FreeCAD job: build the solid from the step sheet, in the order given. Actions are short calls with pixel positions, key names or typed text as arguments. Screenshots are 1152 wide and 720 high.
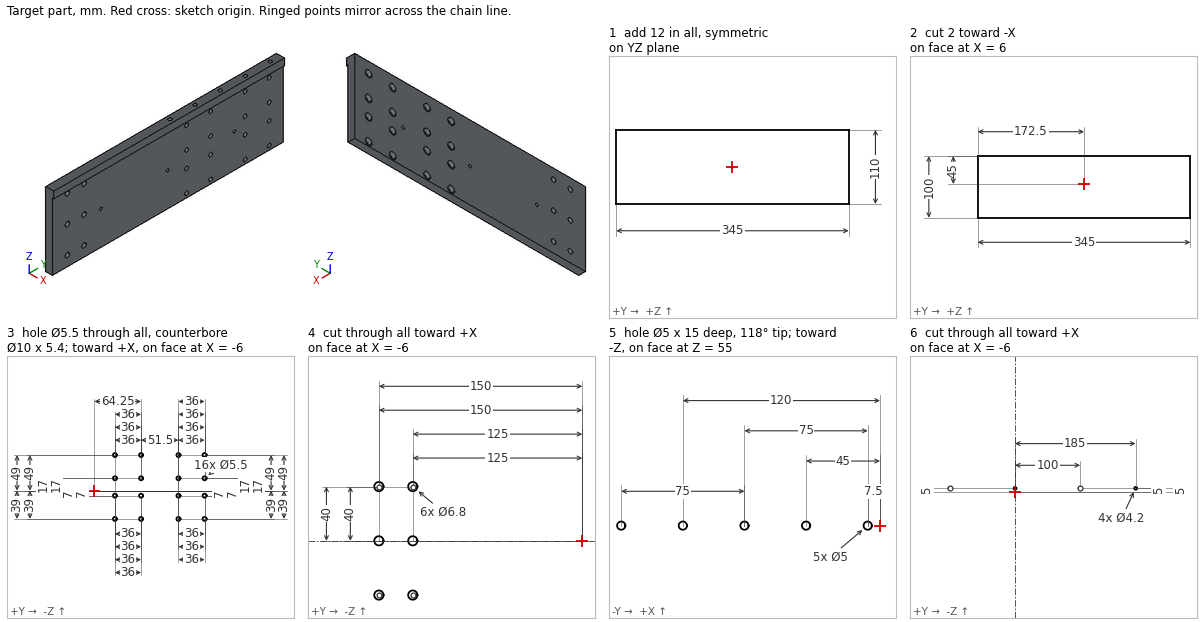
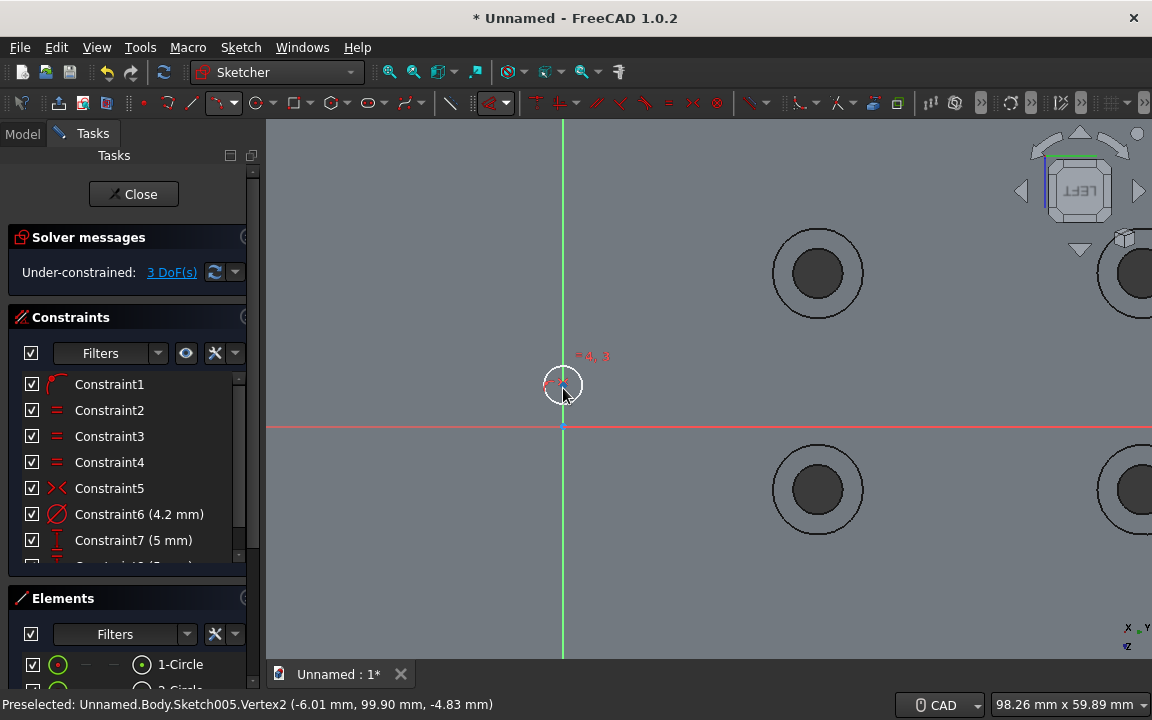
click(563, 385)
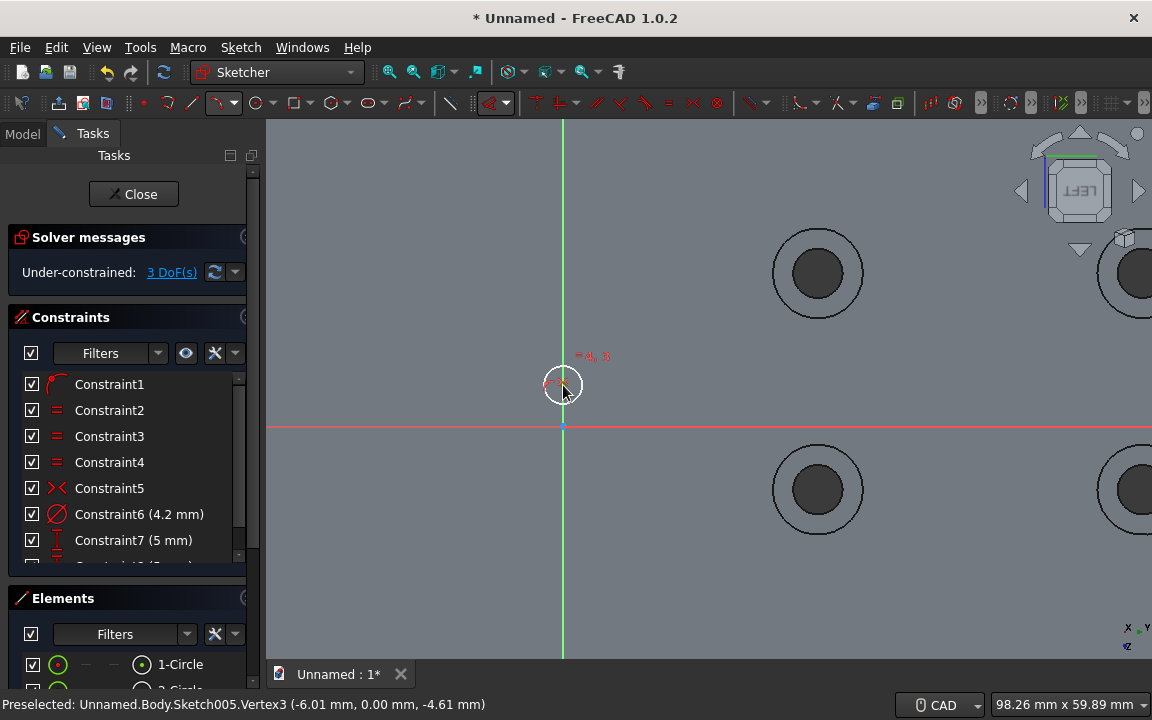
key(i)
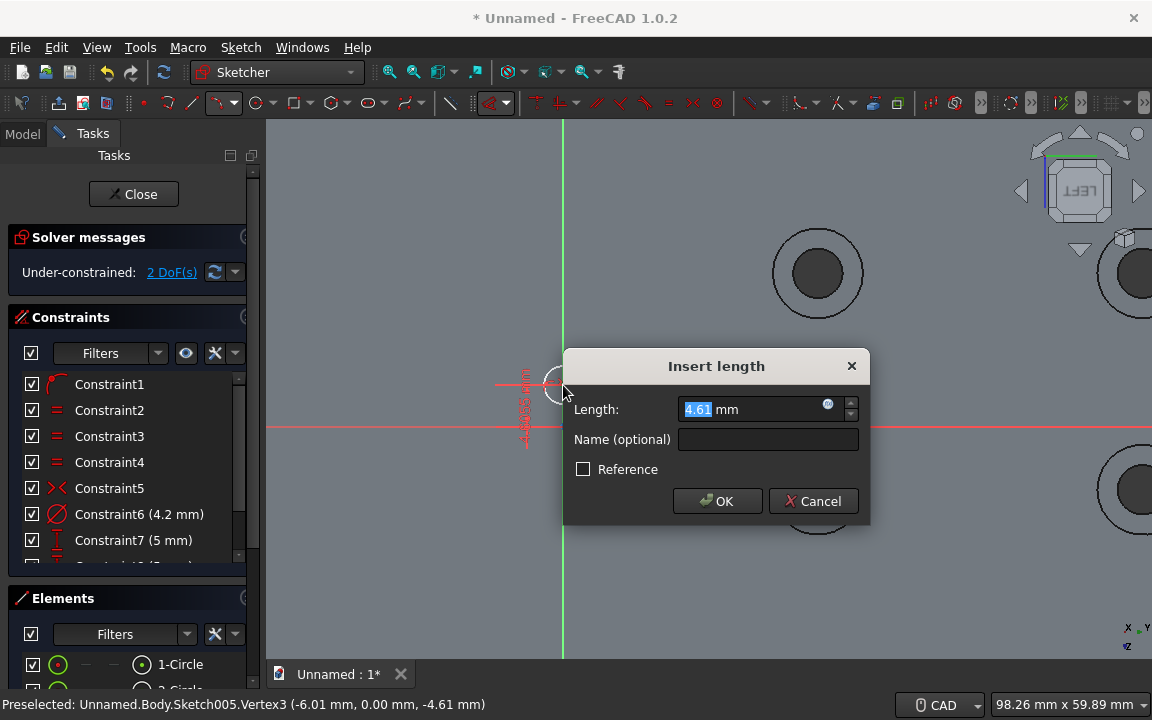
text(5)
key(Return)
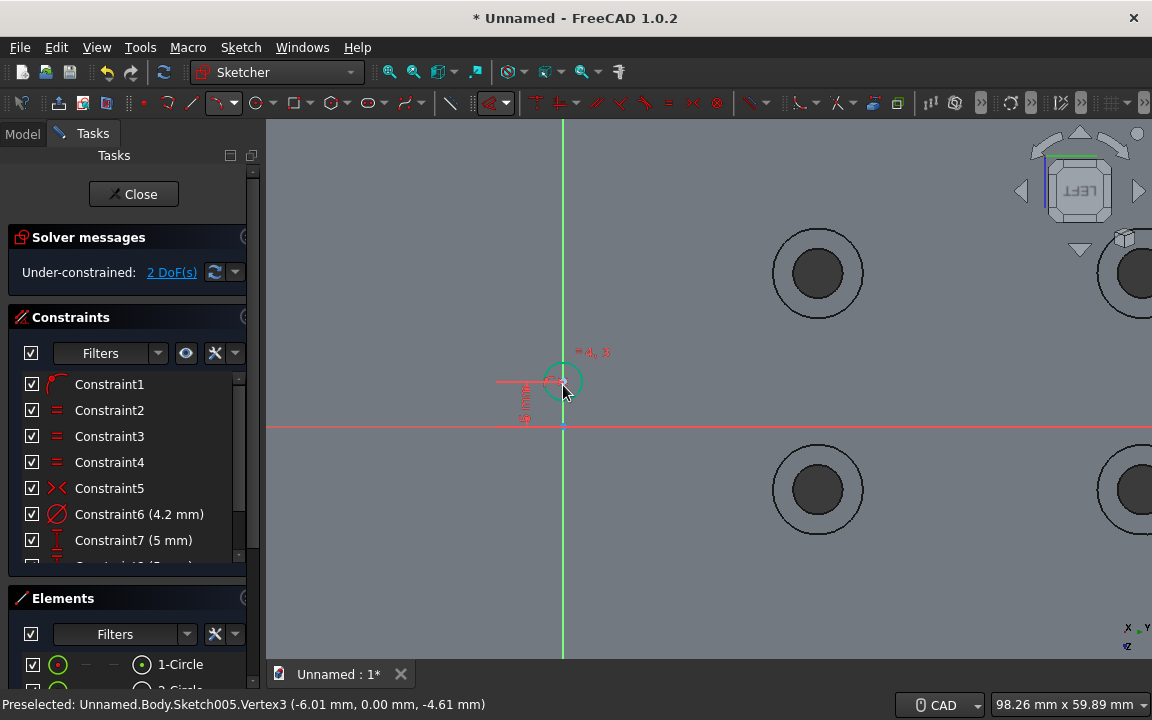
scroll(563, 388, down, 8)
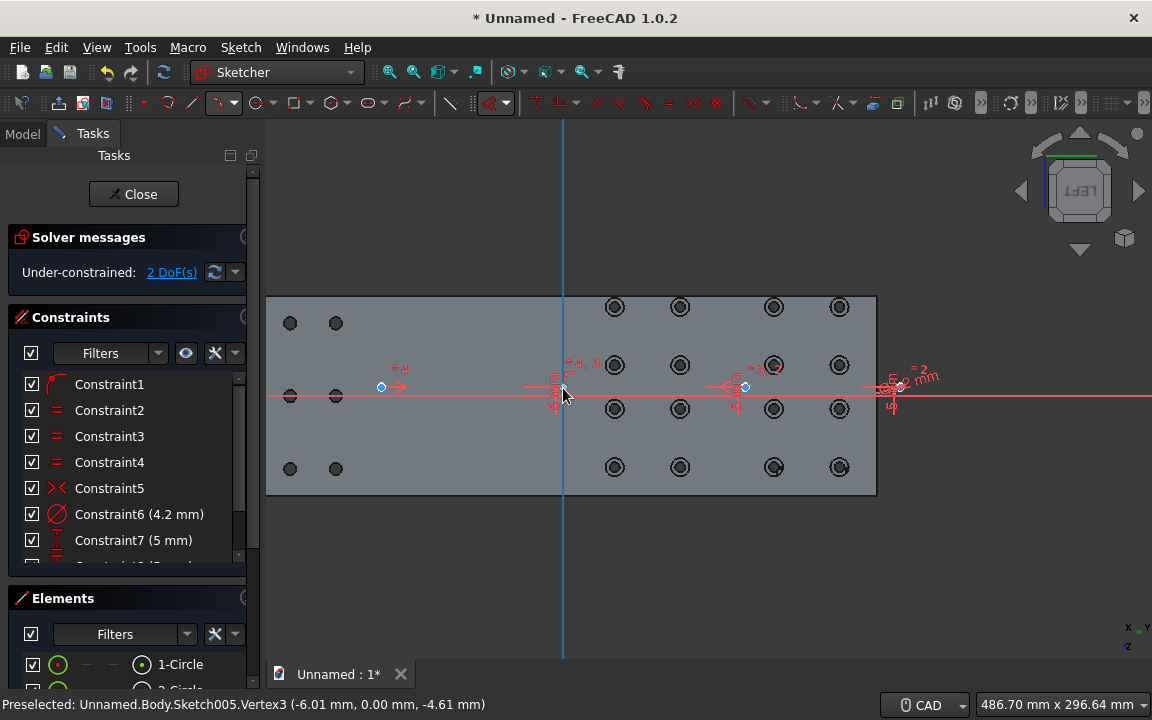
click(900, 387)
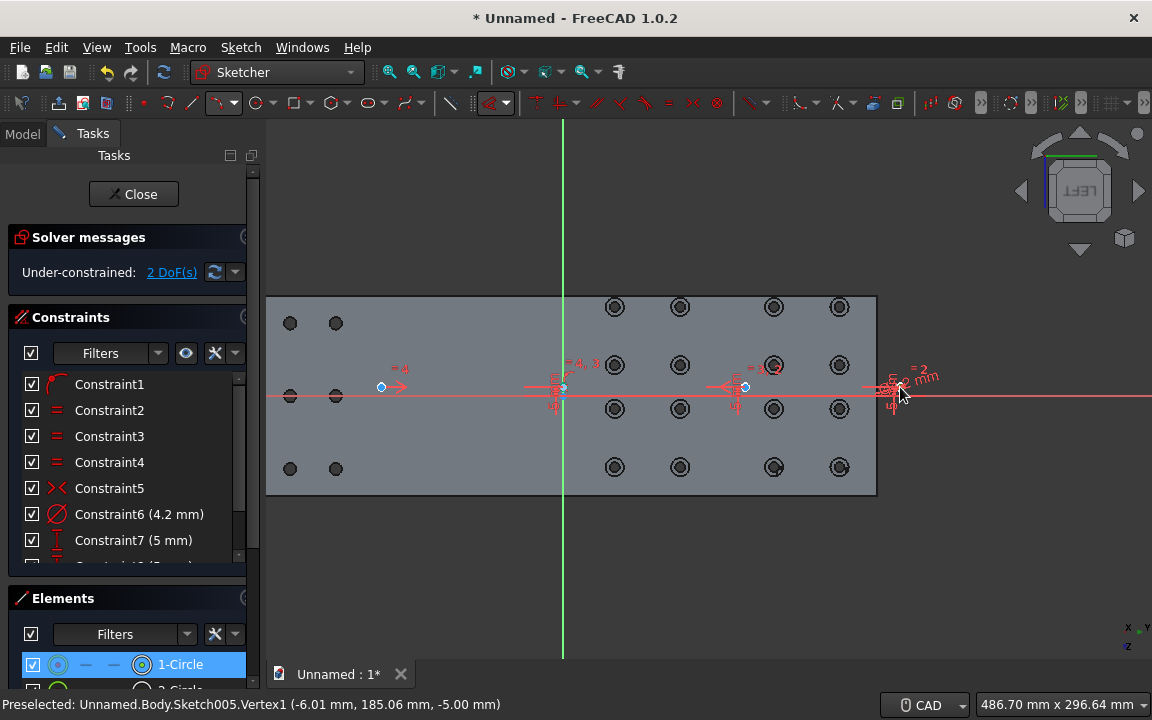
click(508, 104)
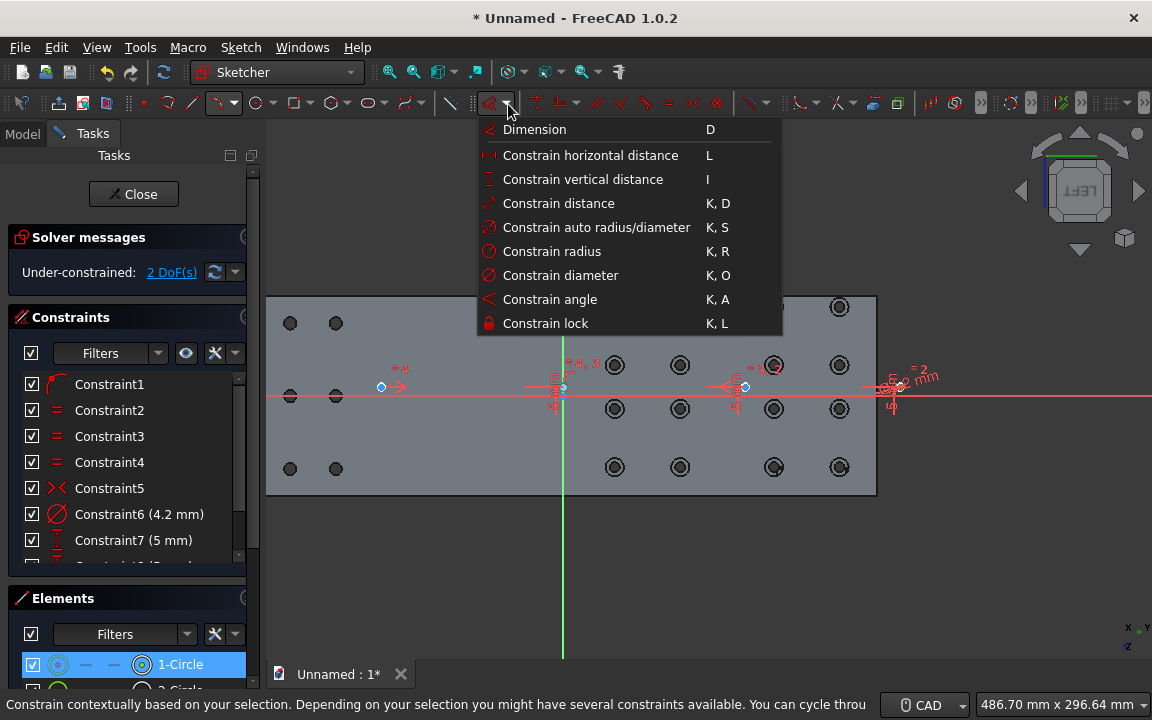
click(630, 155)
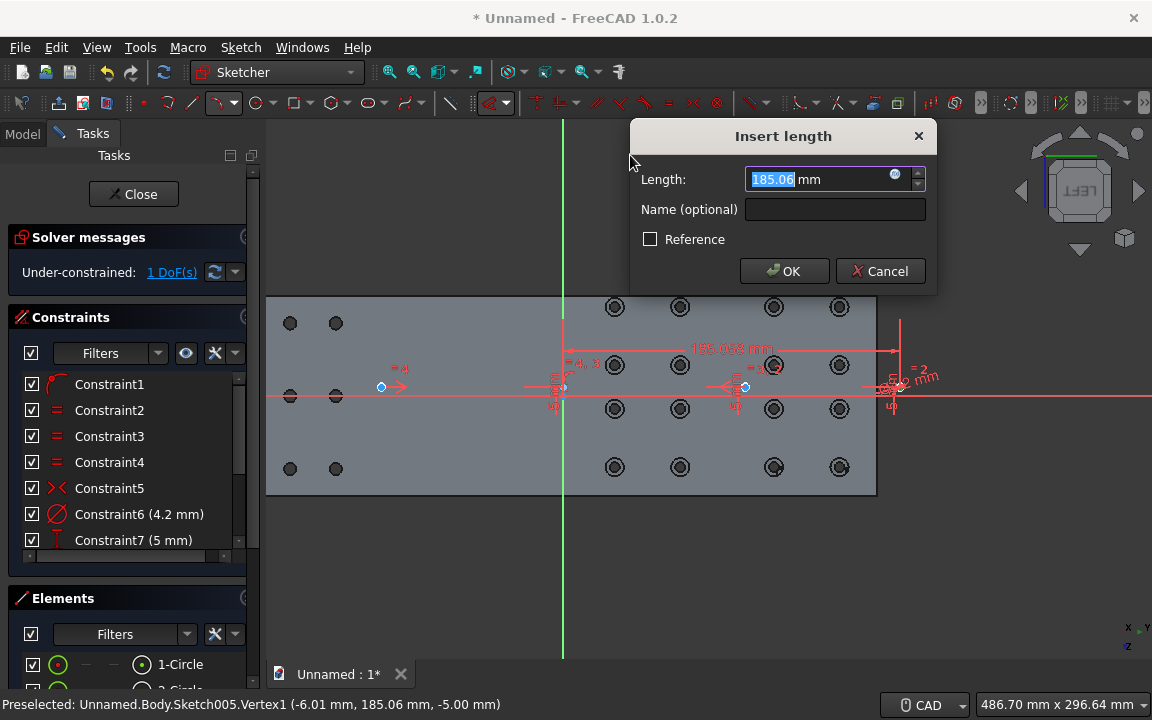
text(185)
key(Return)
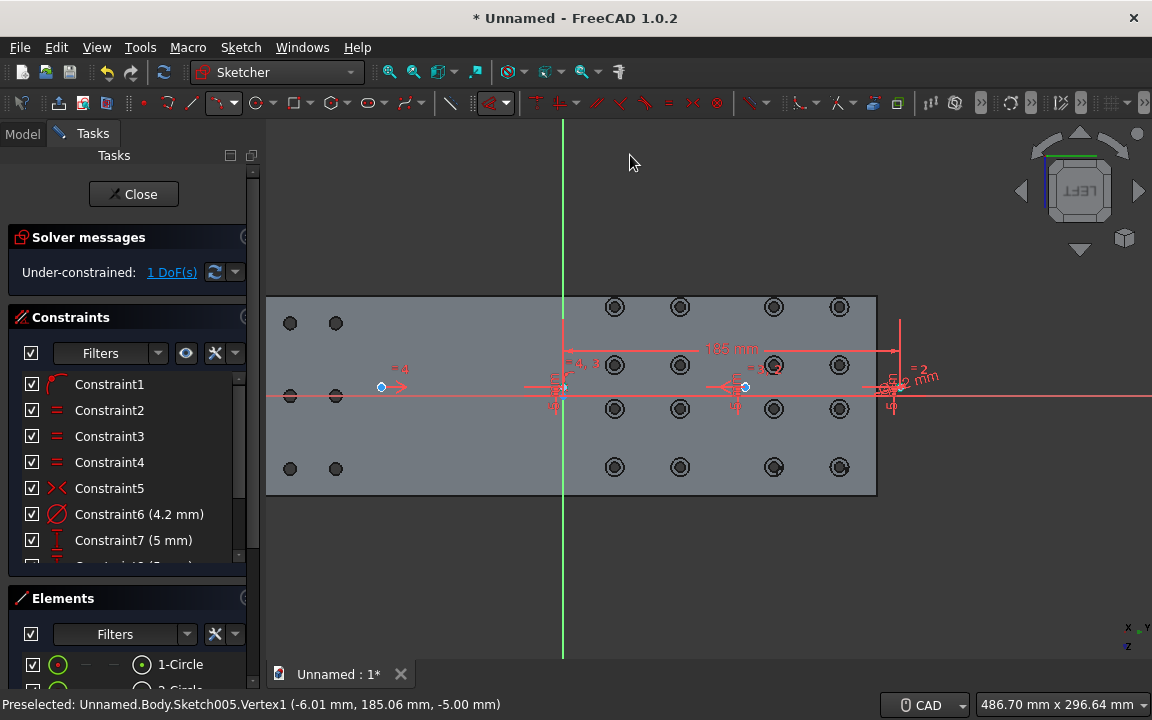
click(745, 387)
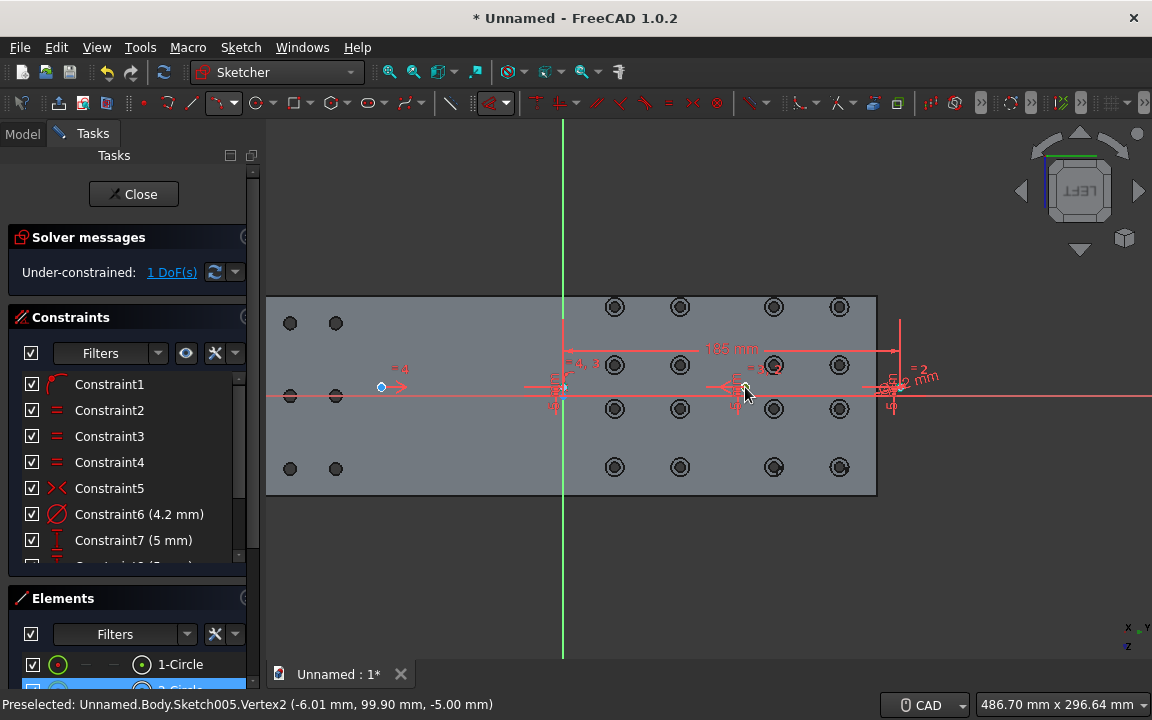
click(508, 104)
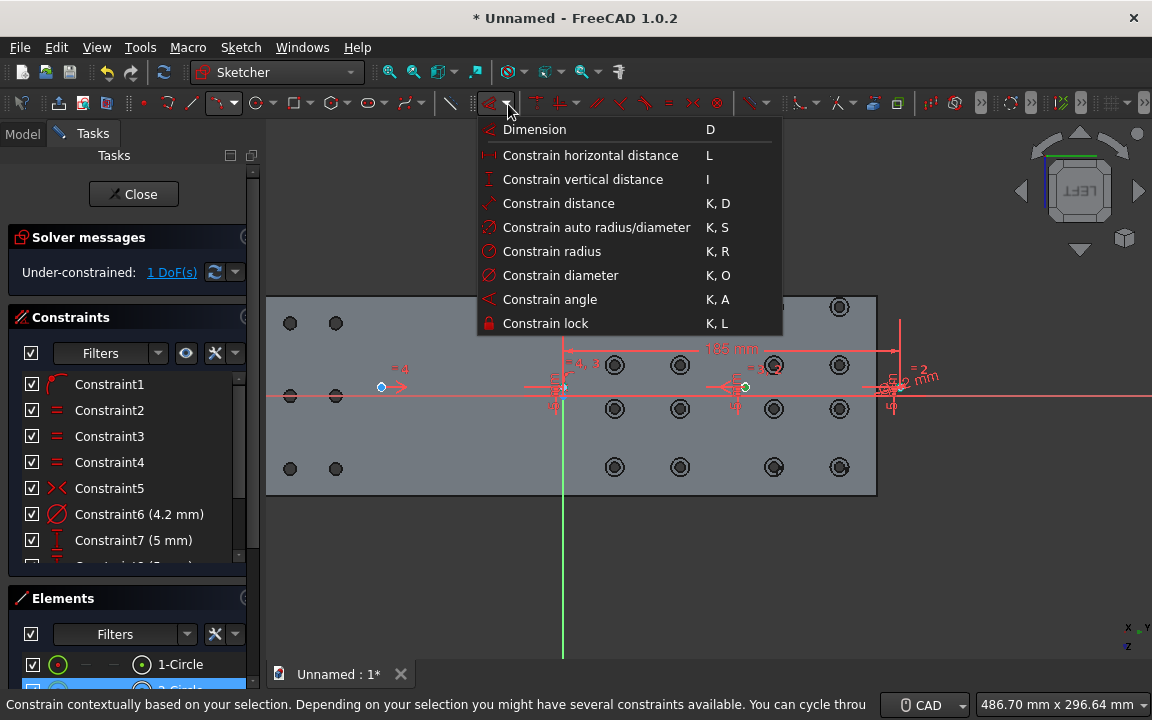
click(630, 155)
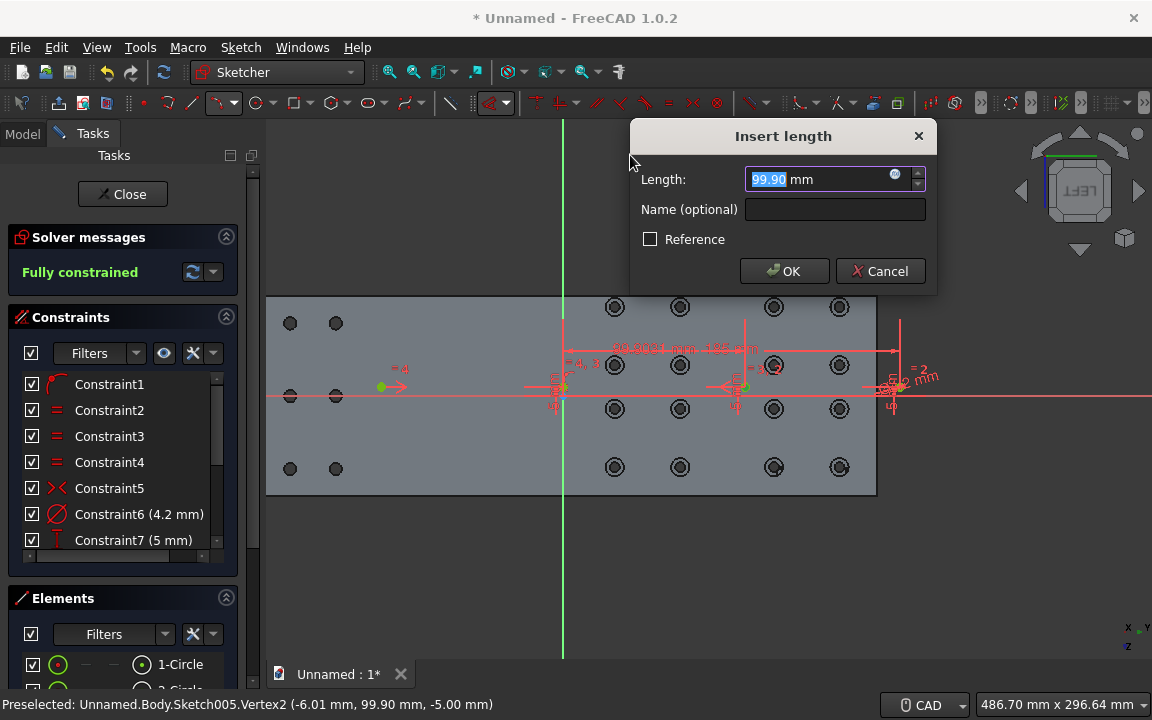
text(100)
key(Return)